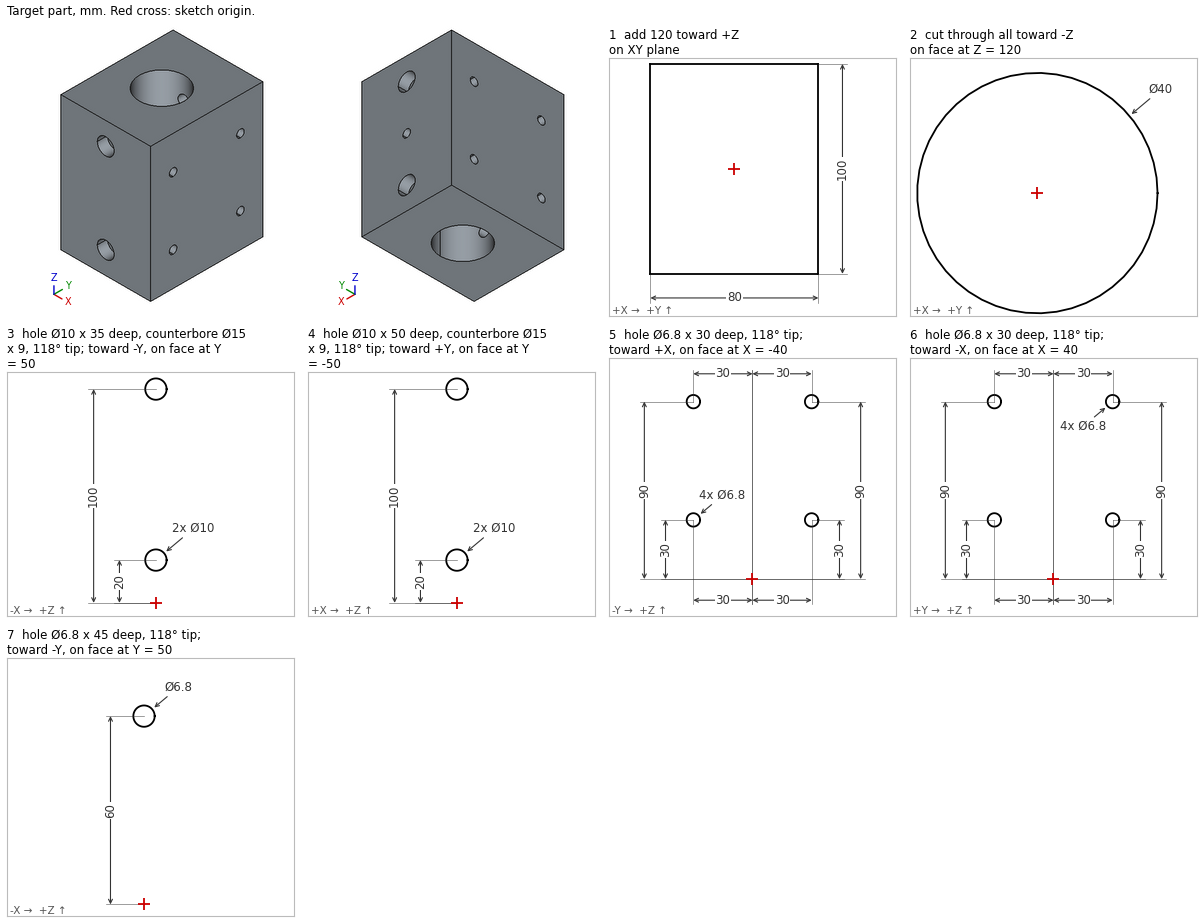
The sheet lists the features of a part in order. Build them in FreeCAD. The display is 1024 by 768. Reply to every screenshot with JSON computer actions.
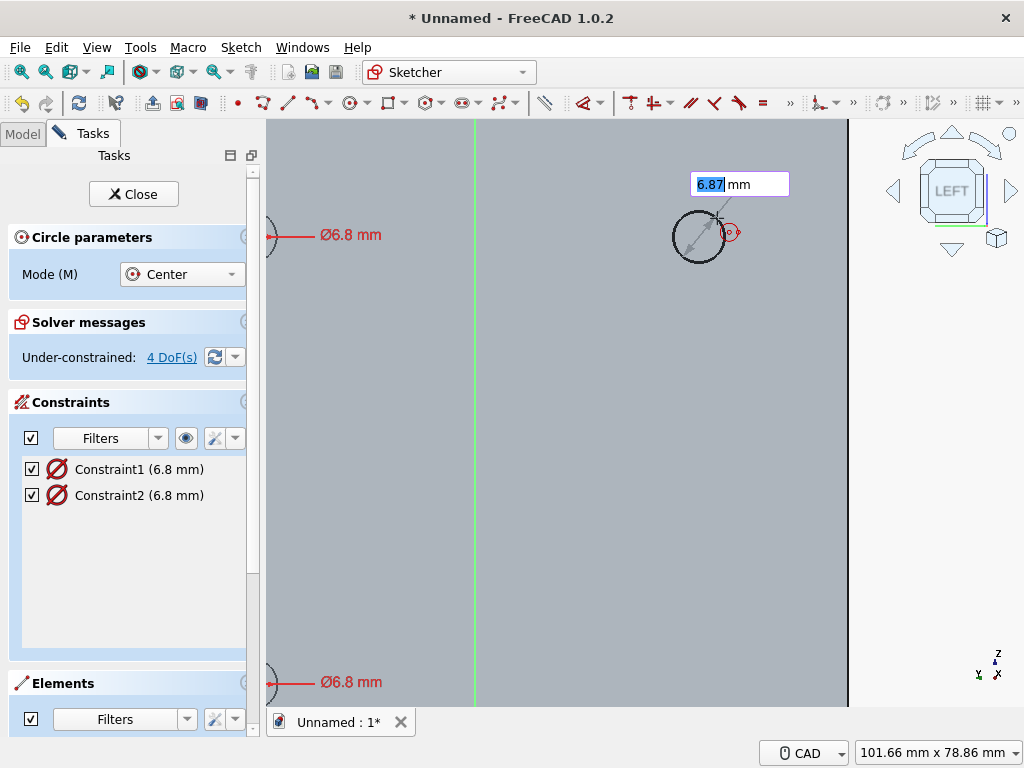
{"action": "type", "text": "6.8"}
{"action": "key", "text": "Return"}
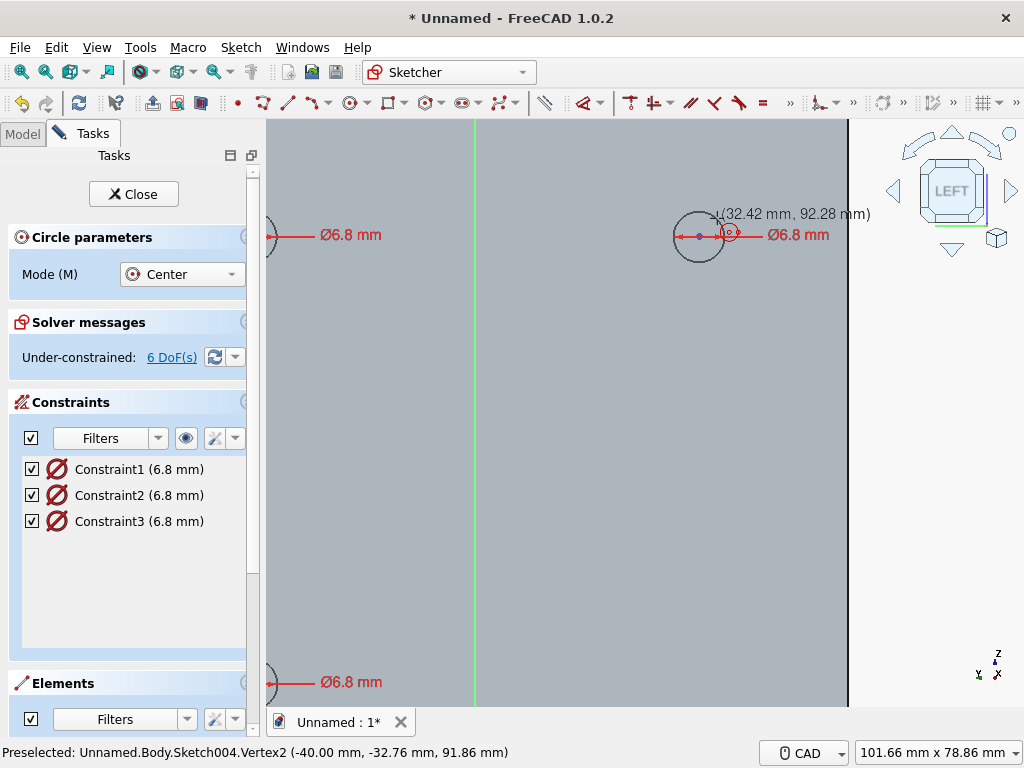
{"action": "scroll", "coordinate": [700, 236], "scroll_direction": "down", "scroll_amount": 3}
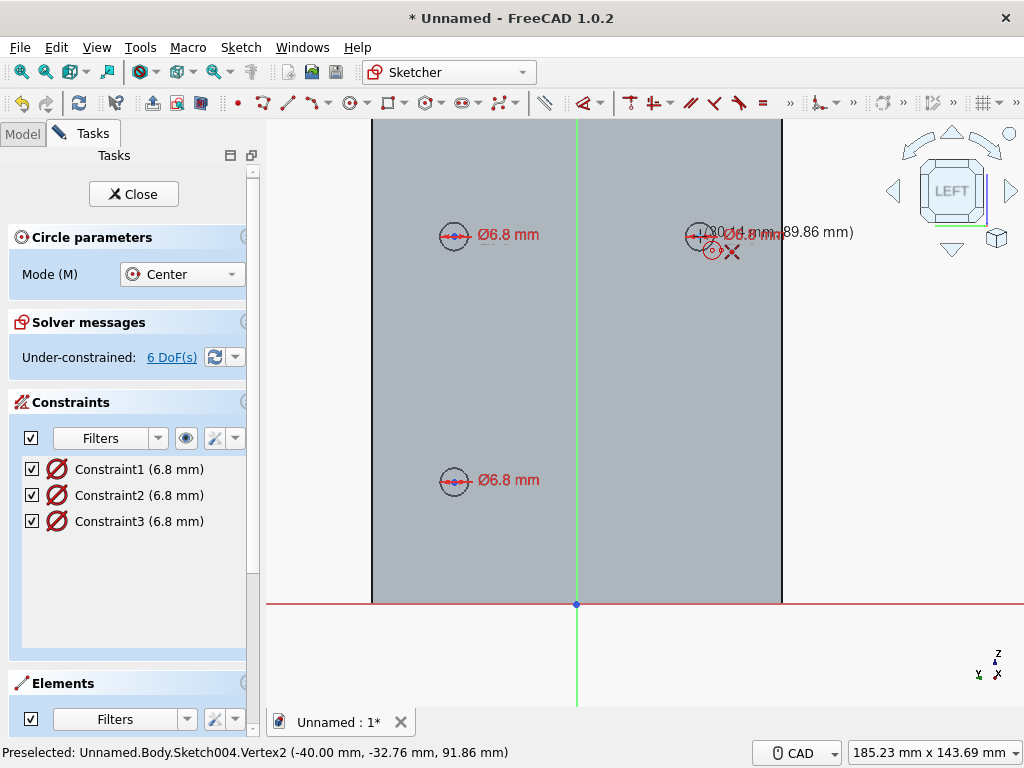
{"action": "scroll", "coordinate": [700, 482], "scroll_direction": "up", "scroll_amount": 3}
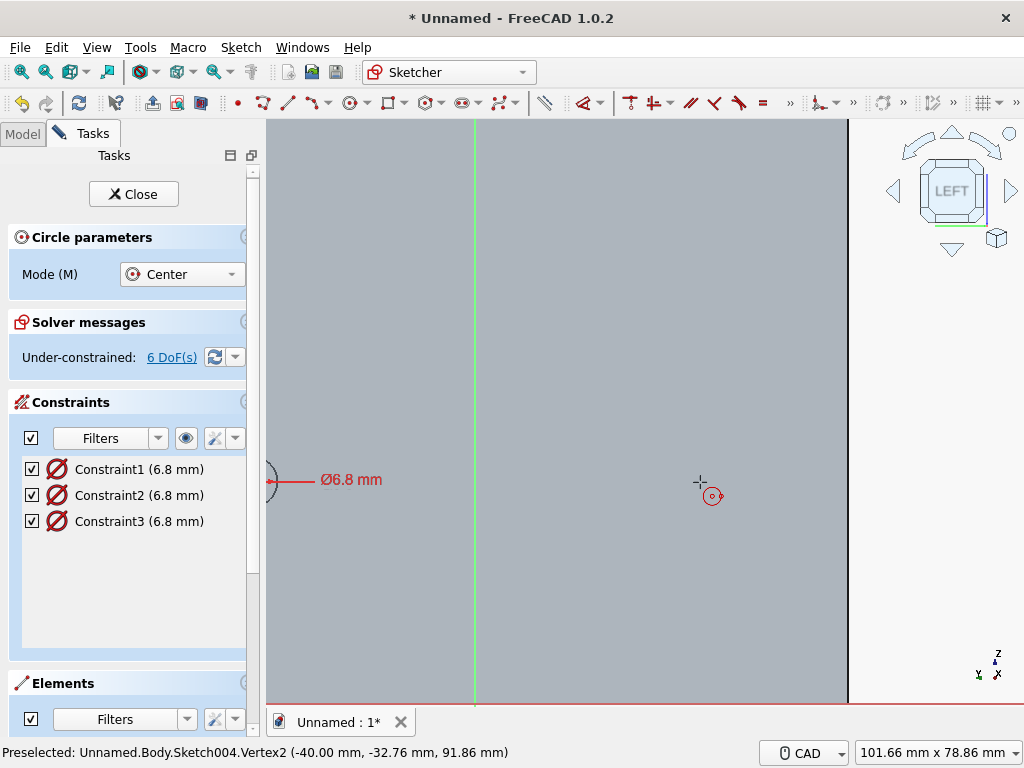
{"action": "left_click", "coordinate": [699, 481]}
{"action": "mouse_move", "coordinate": [717, 463]}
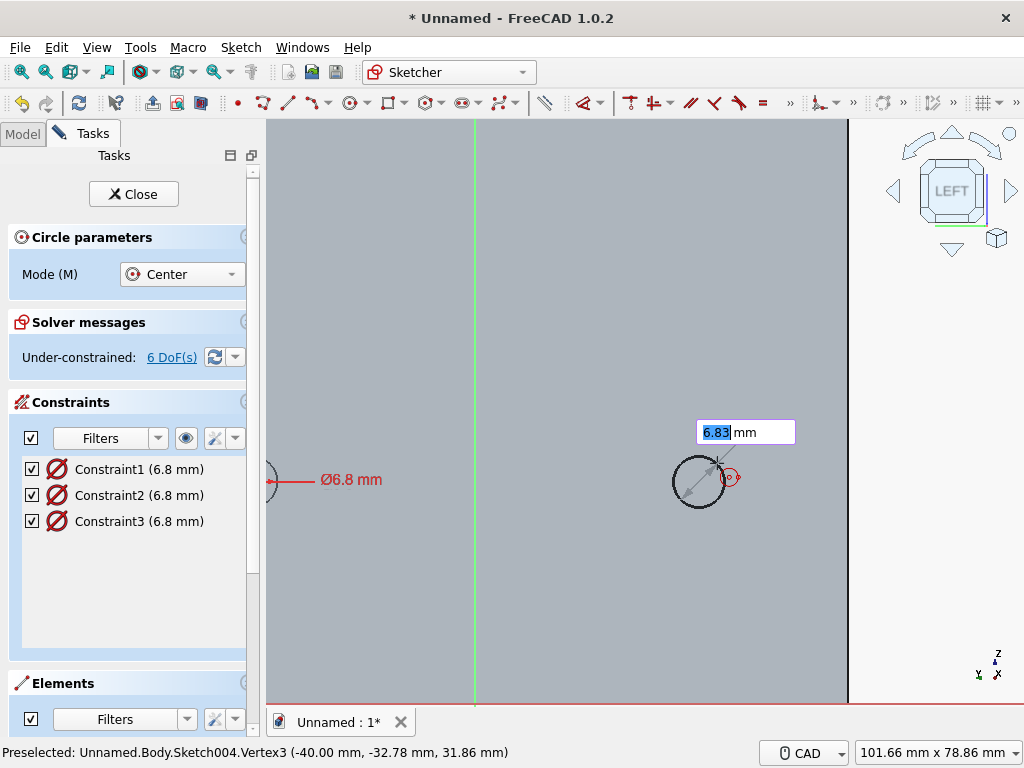
{"action": "type", "text": "6.8"}
{"action": "key", "text": "Return"}
{"action": "key", "text": "Escape"}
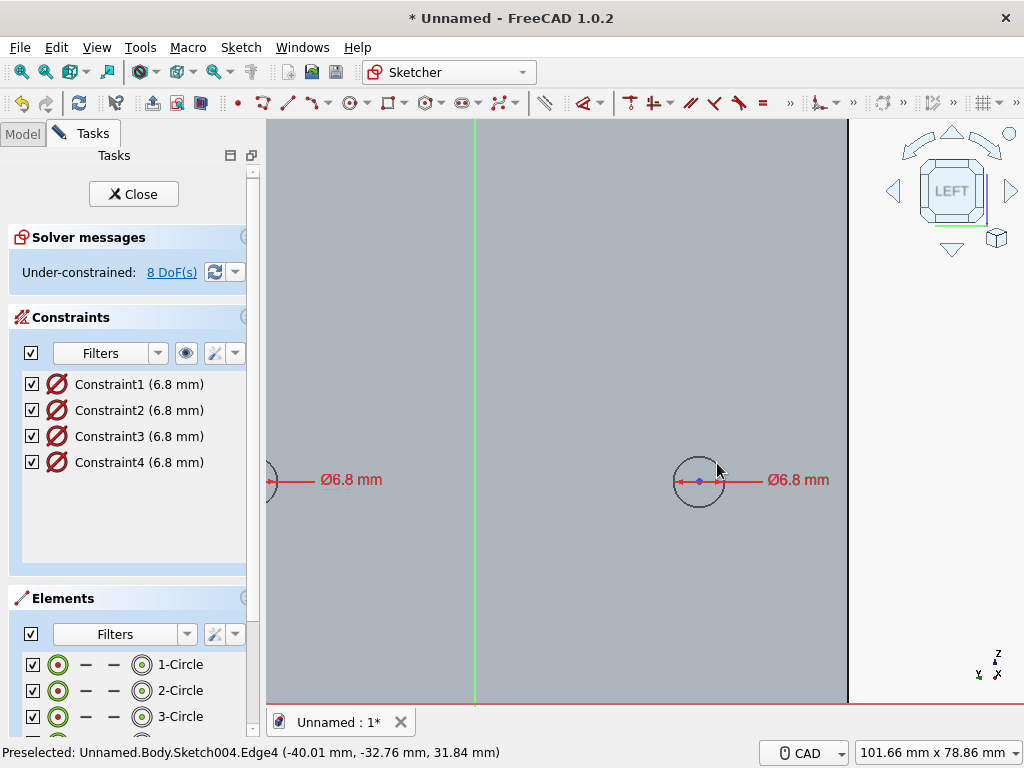
{"action": "left_click", "coordinate": [584, 104]}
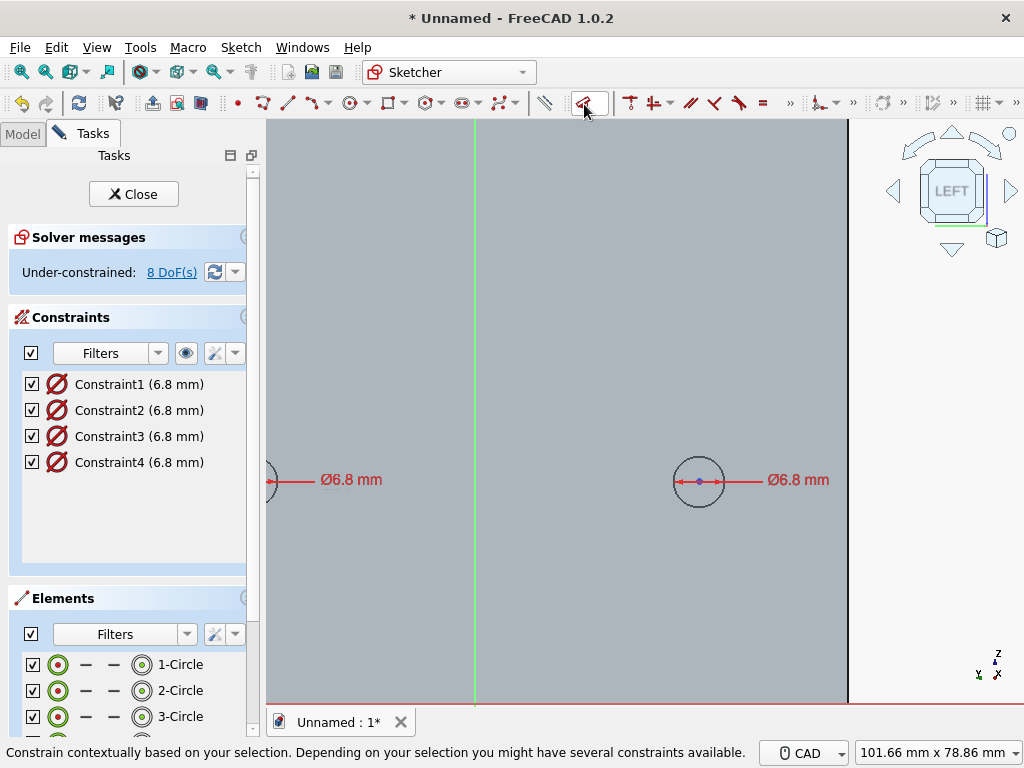
{"action": "scroll", "coordinate": [700, 482], "scroll_direction": "down", "scroll_amount": 3}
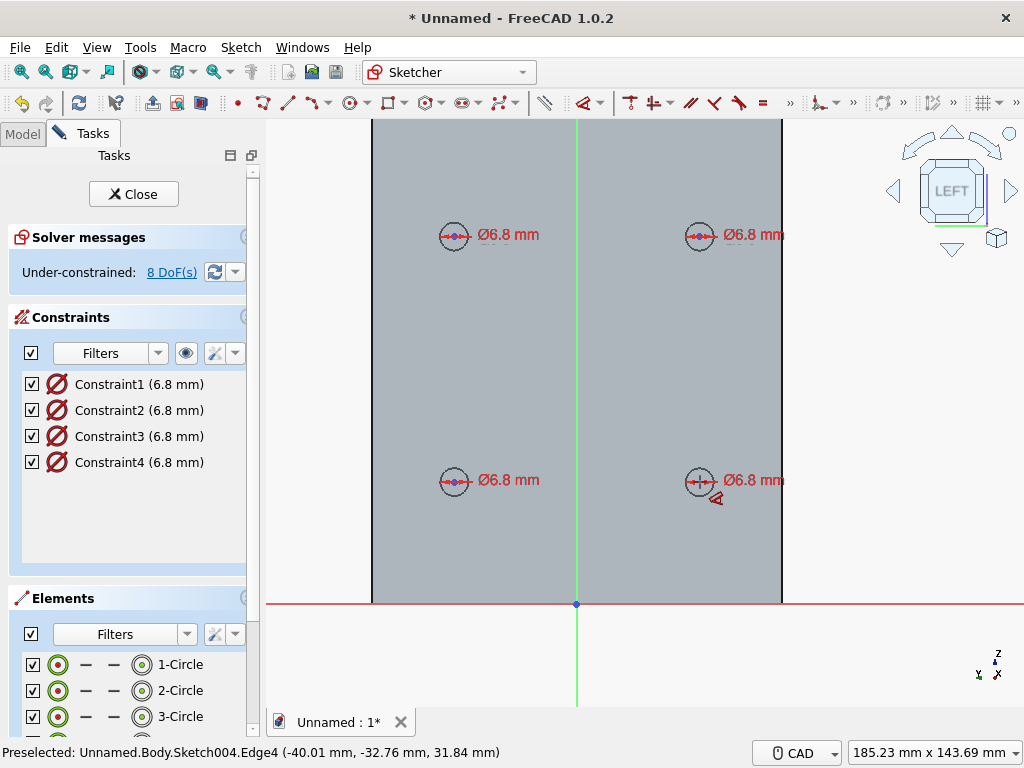
{"action": "left_click", "coordinate": [454, 482]}
{"action": "left_click", "coordinate": [516, 638]}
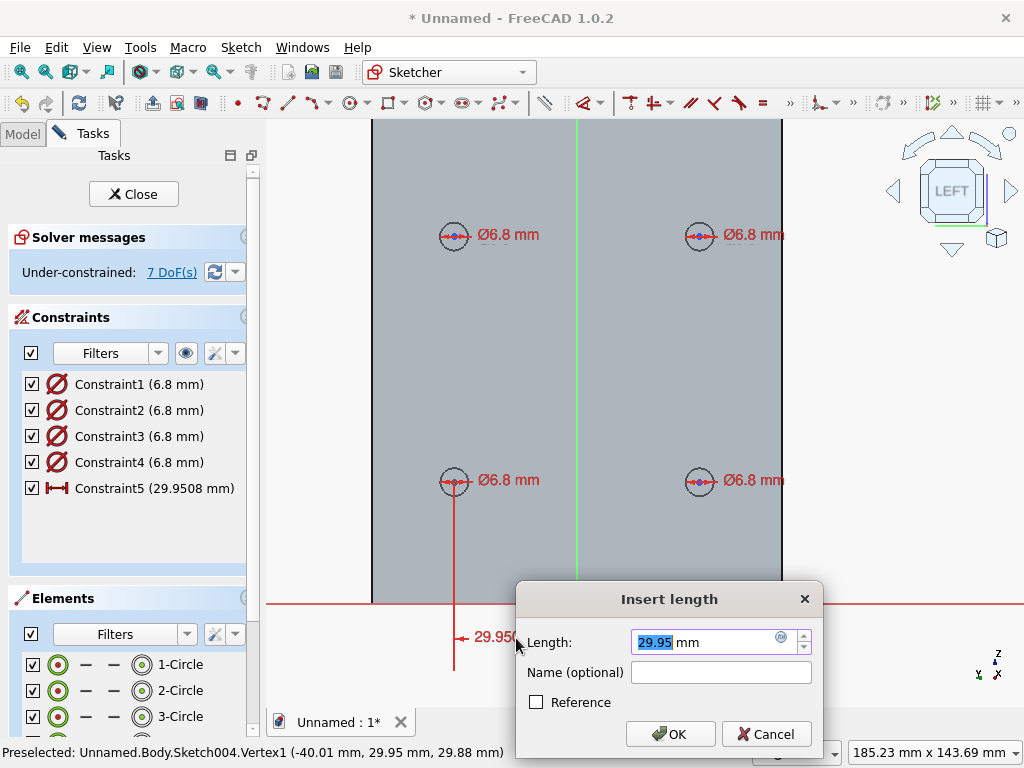
{"action": "type", "text": "30"}
{"action": "key", "text": "Return"}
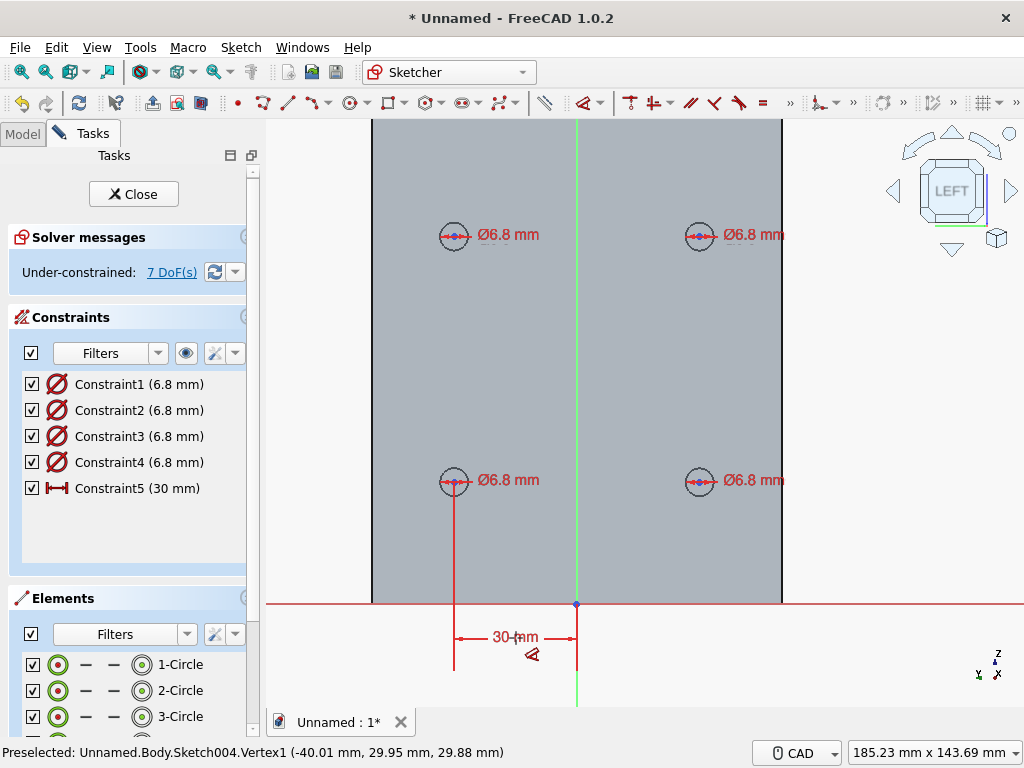
{"action": "left_click", "coordinate": [454, 482]}
{"action": "left_click", "coordinate": [420, 543]}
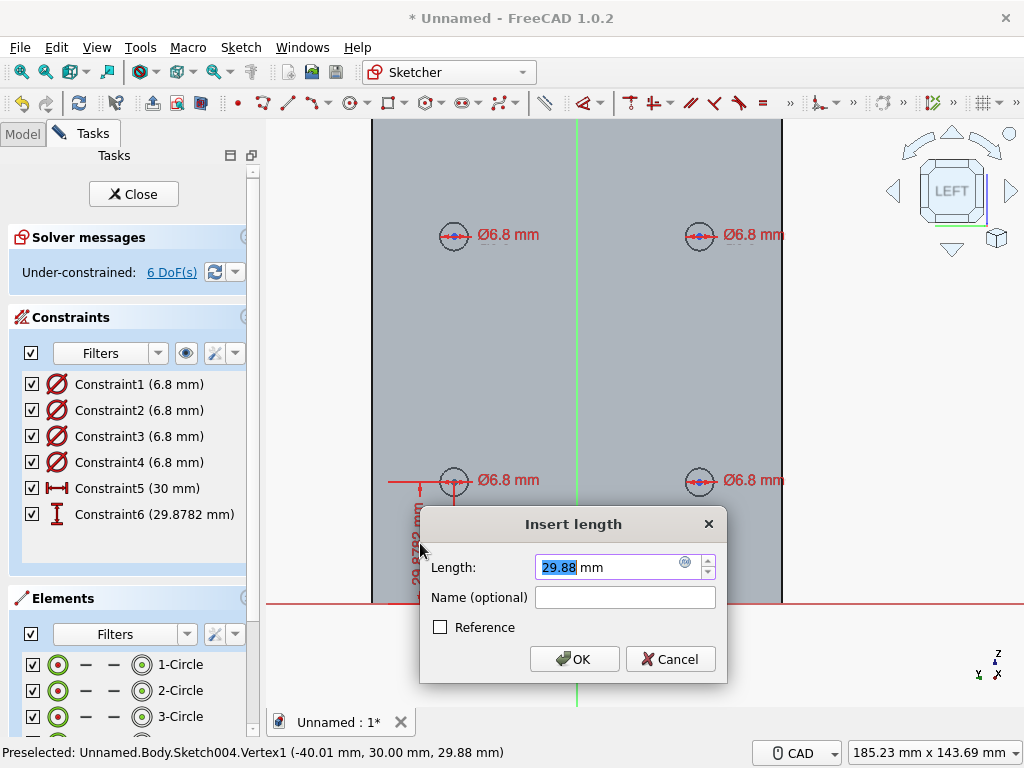
{"action": "type", "text": "30"}
{"action": "key", "text": "Return"}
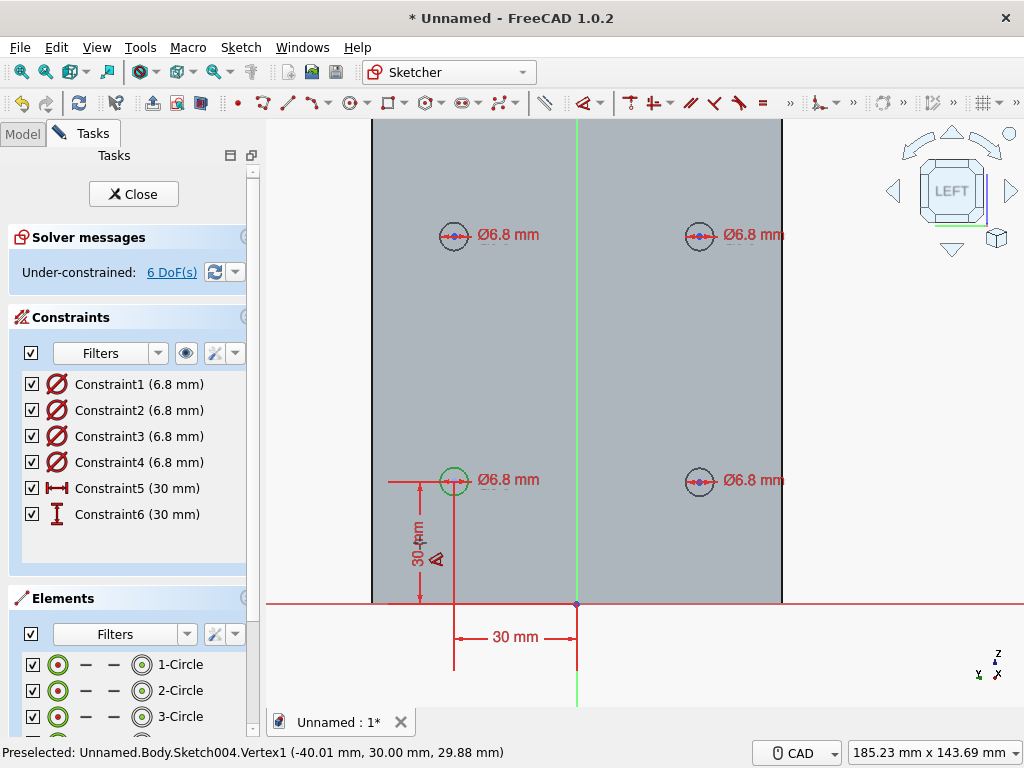
{"action": "left_click", "coordinate": [454, 237]}
{"action": "left_click", "coordinate": [515, 203]}